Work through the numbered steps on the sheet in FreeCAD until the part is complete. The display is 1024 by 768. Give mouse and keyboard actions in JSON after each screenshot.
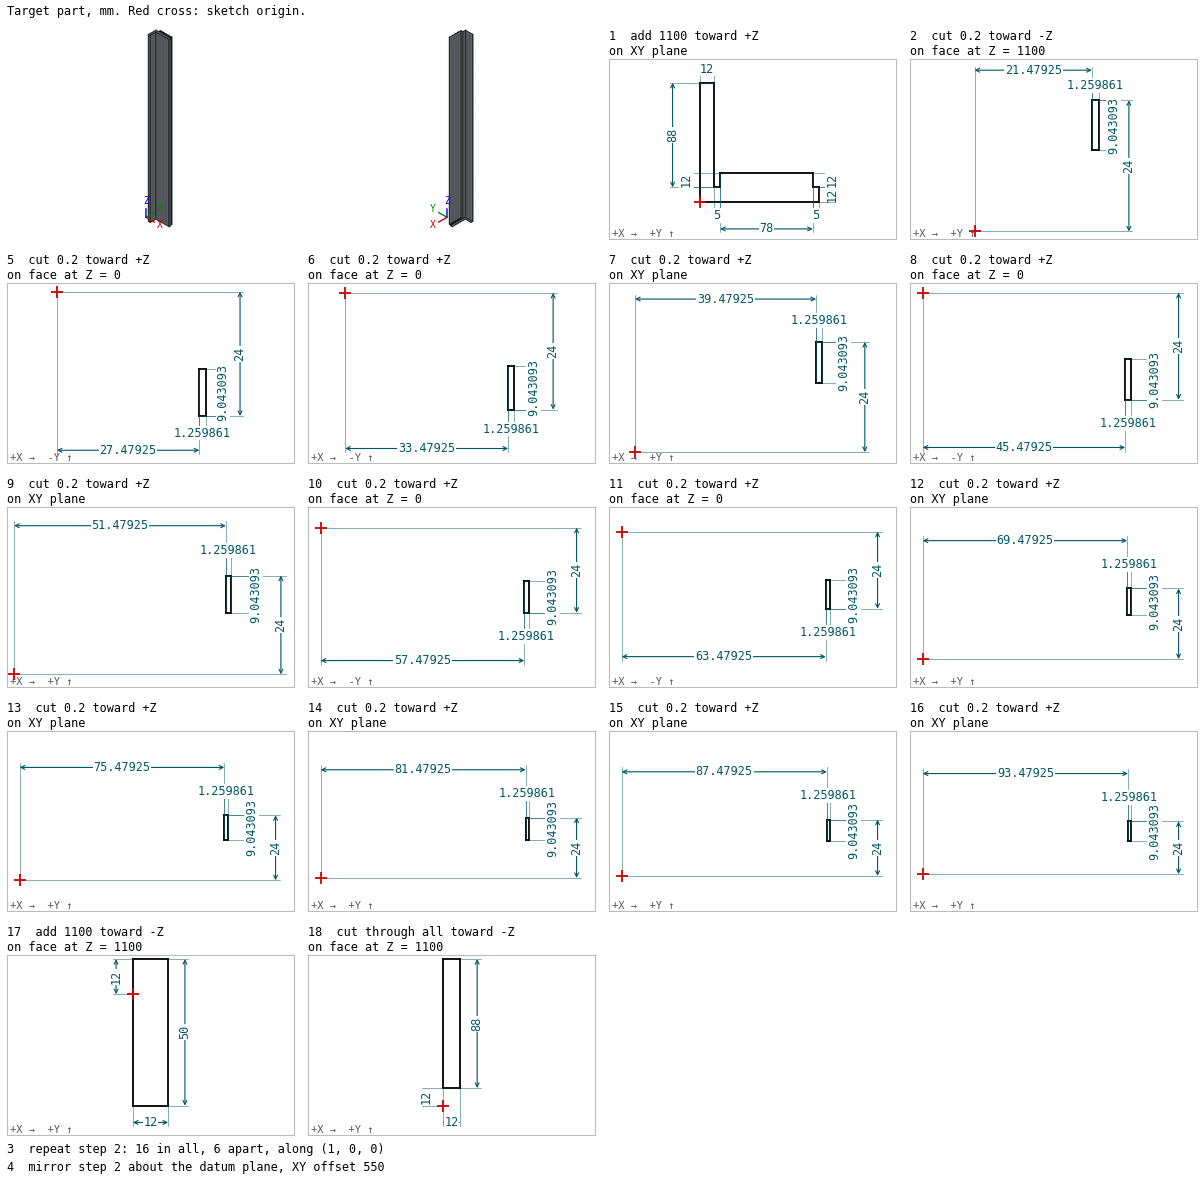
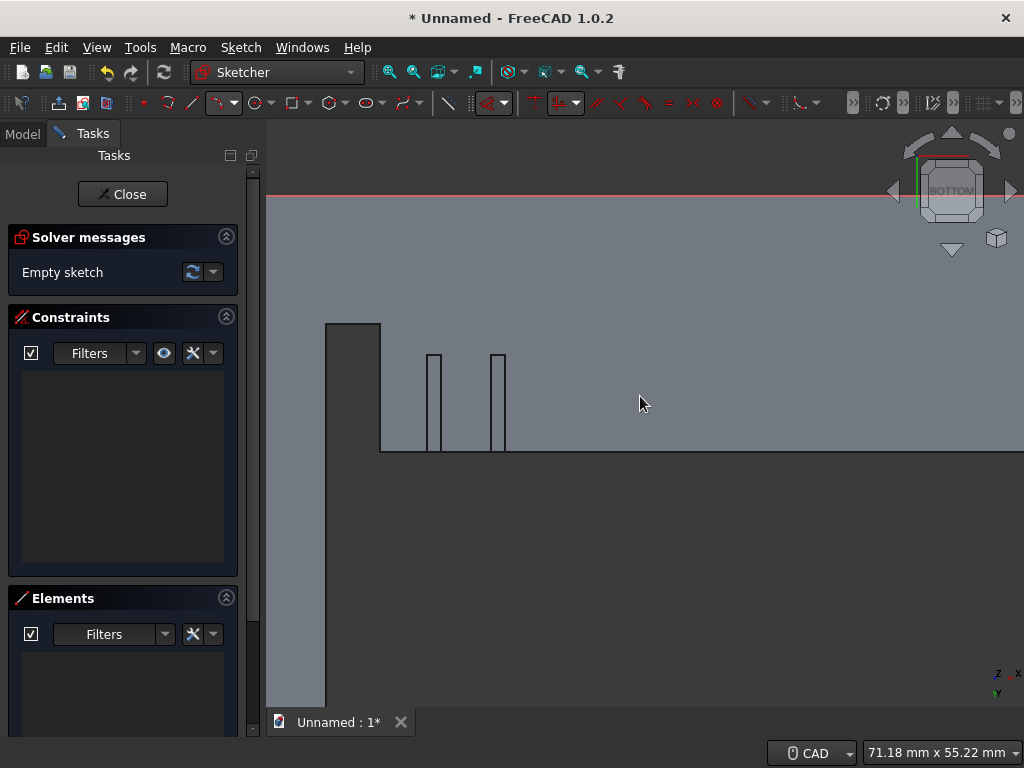
{"action": "scroll", "coordinate": [557, 400], "scroll_direction": "up", "scroll_amount": 7}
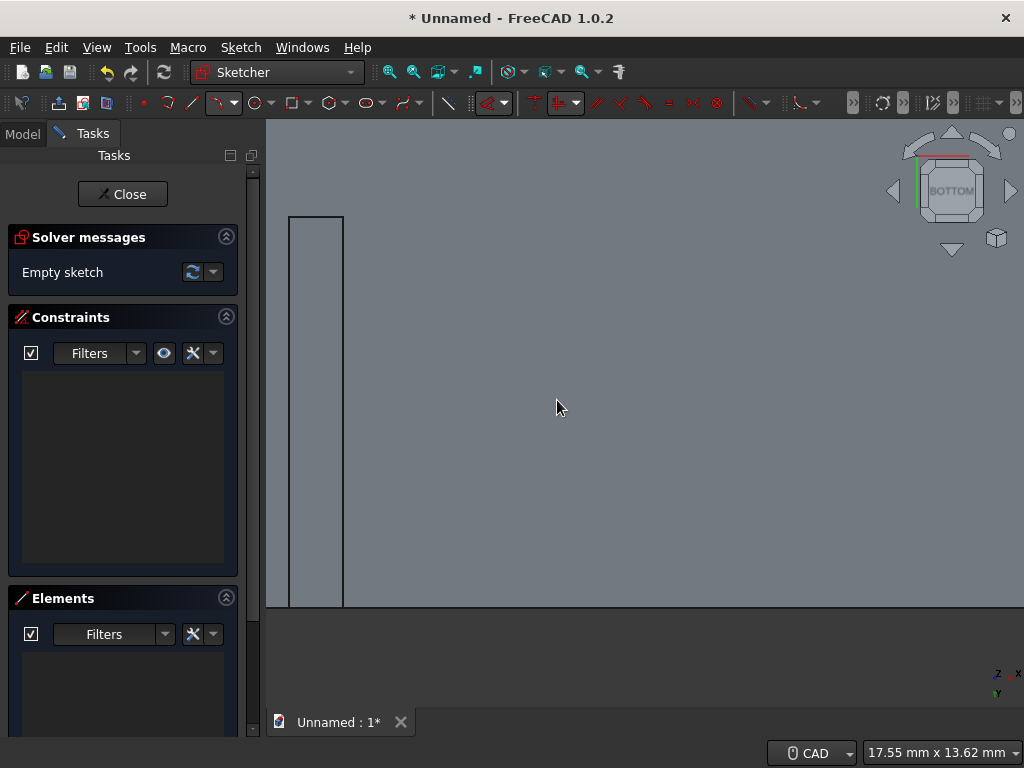
{"action": "key", "text": "g r"}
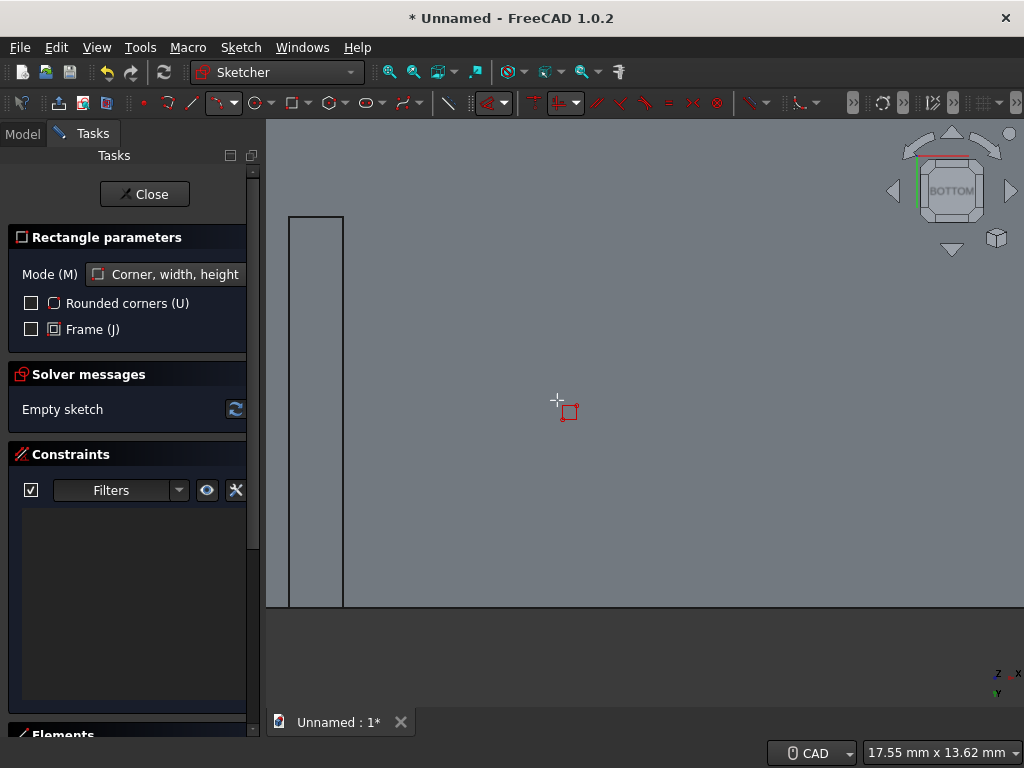
{"action": "left_click", "coordinate": [548, 217]}
{"action": "mouse_move", "coordinate": [602, 608]}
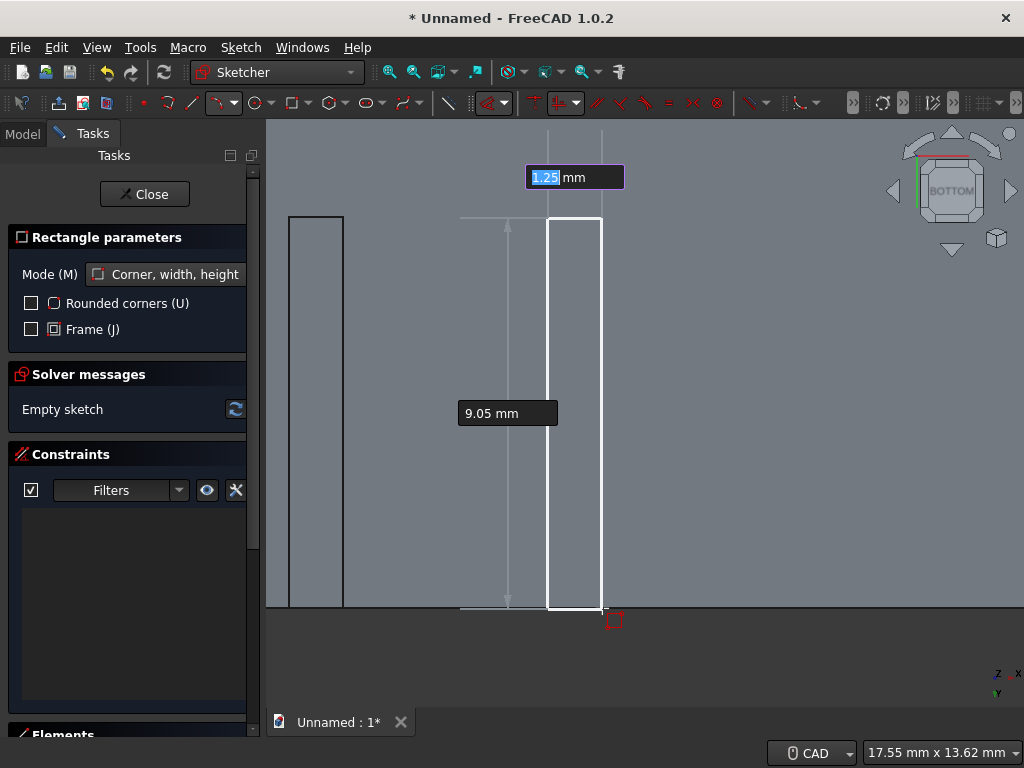
{"action": "type", "text": "1.259861"}
{"action": "key", "text": "Tab"}
{"action": "type", "text": "9.043093"}
{"action": "key", "text": "Return"}
{"action": "key", "text": "Escape"}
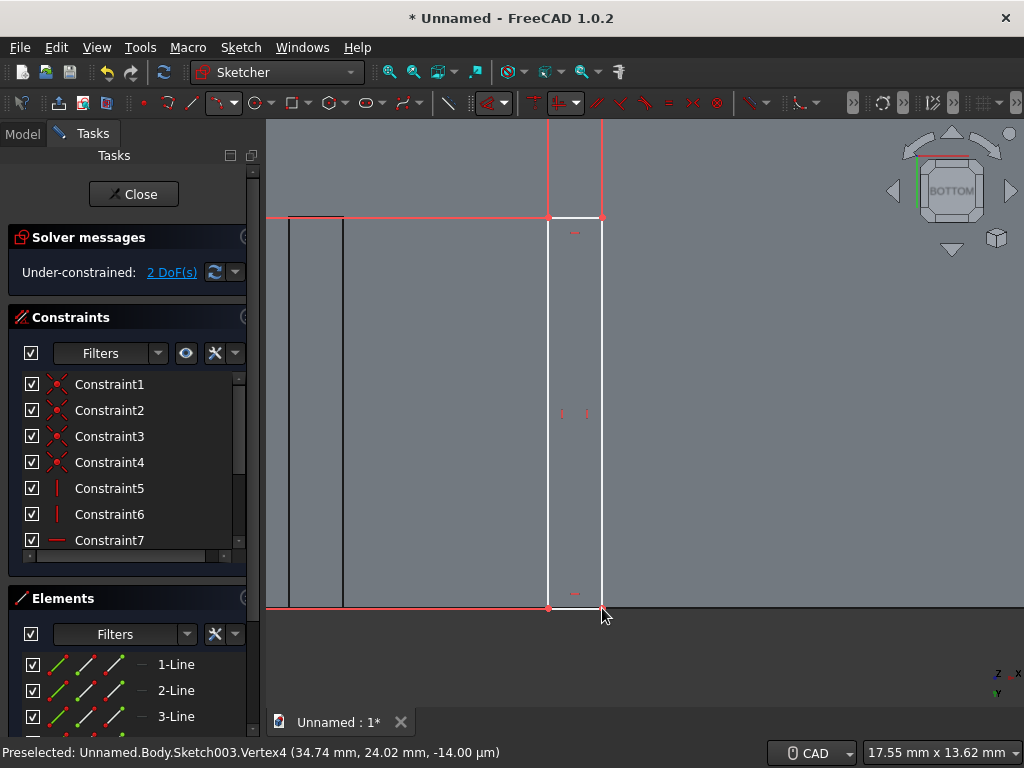
{"action": "left_click", "coordinate": [548, 609]}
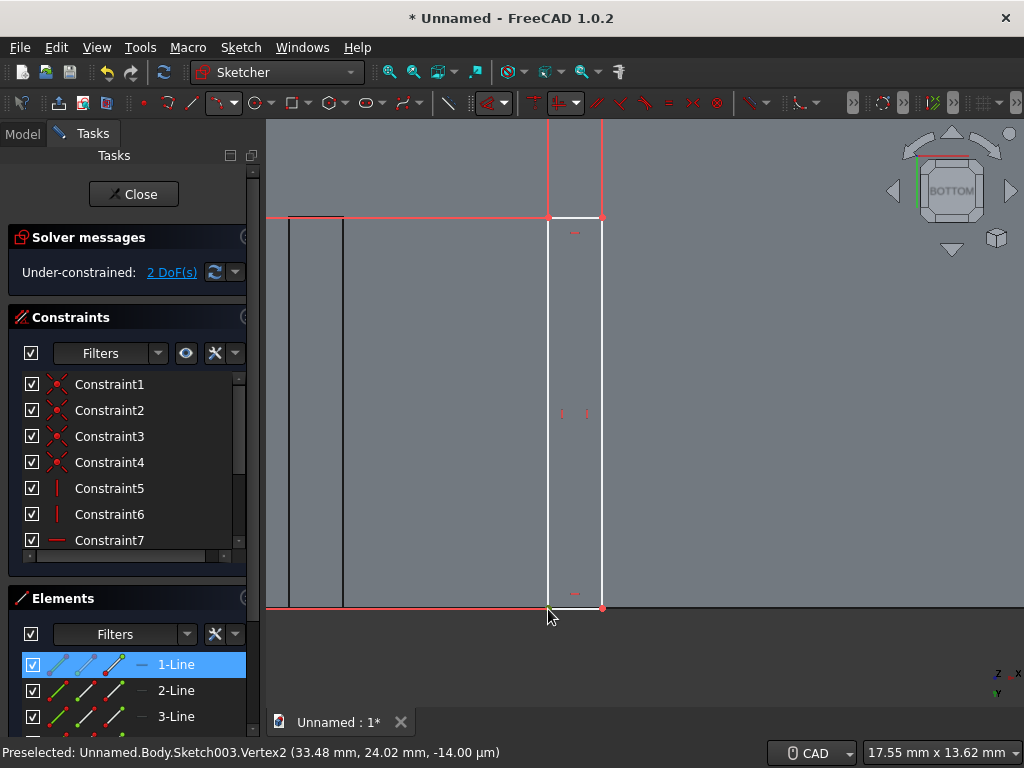
{"action": "left_click", "coordinate": [506, 104]}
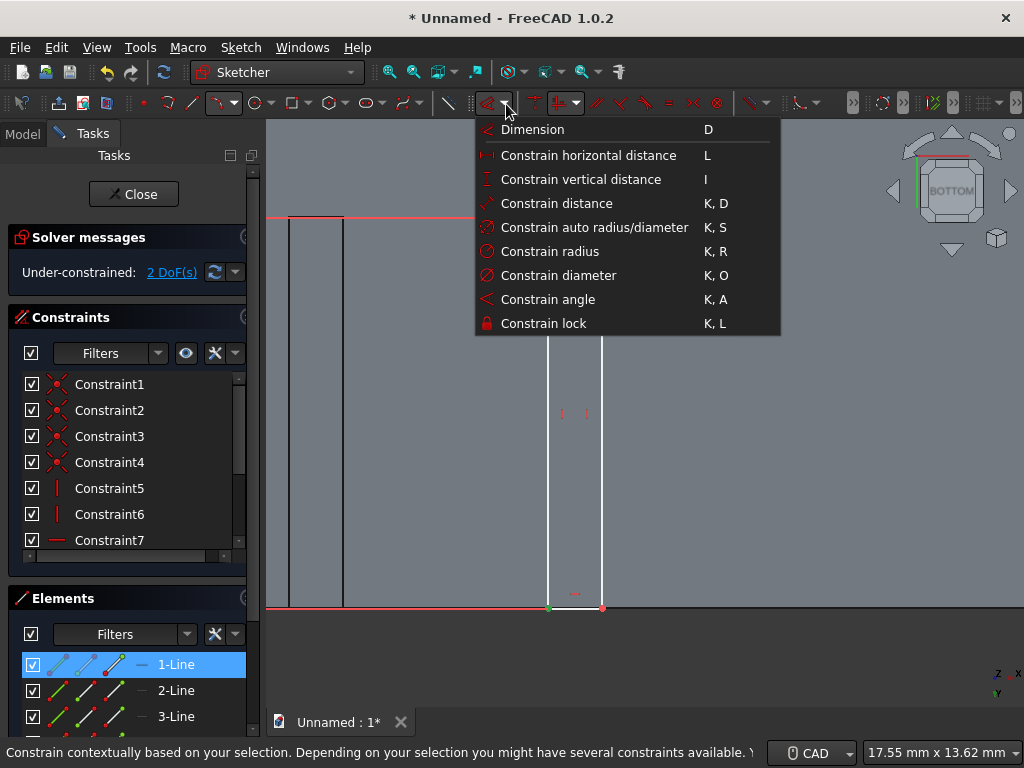
{"action": "left_click", "coordinate": [628, 179]}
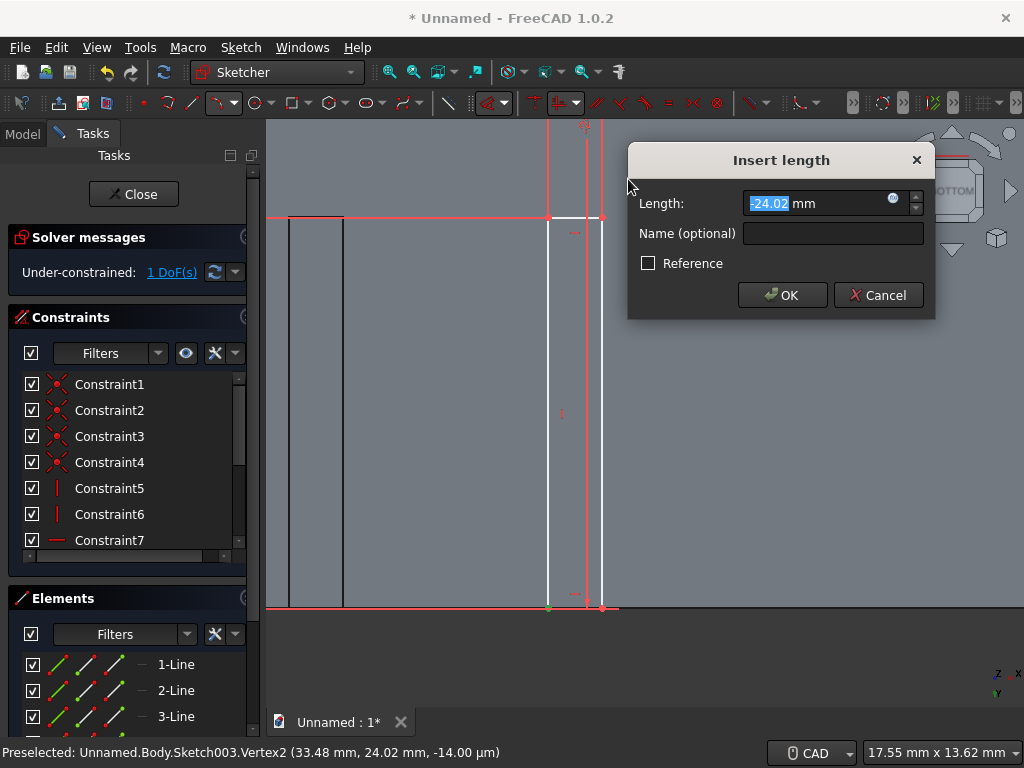
{"action": "type", "text": "-24"}
{"action": "key", "text": "Return"}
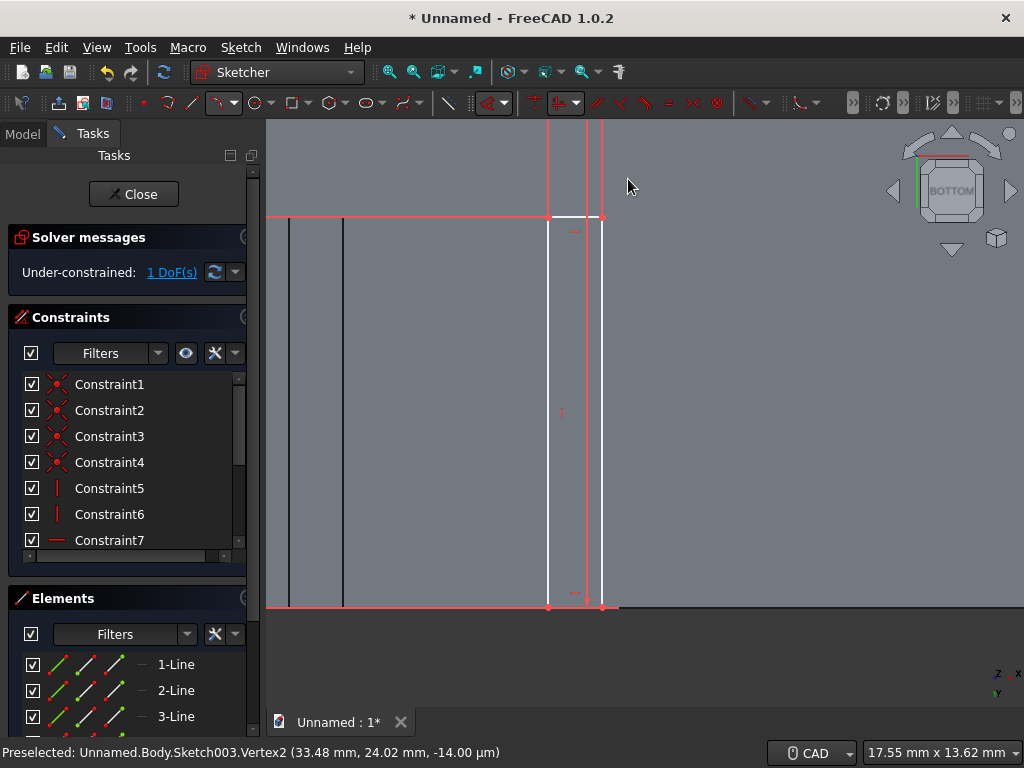
{"action": "left_click", "coordinate": [548, 217]}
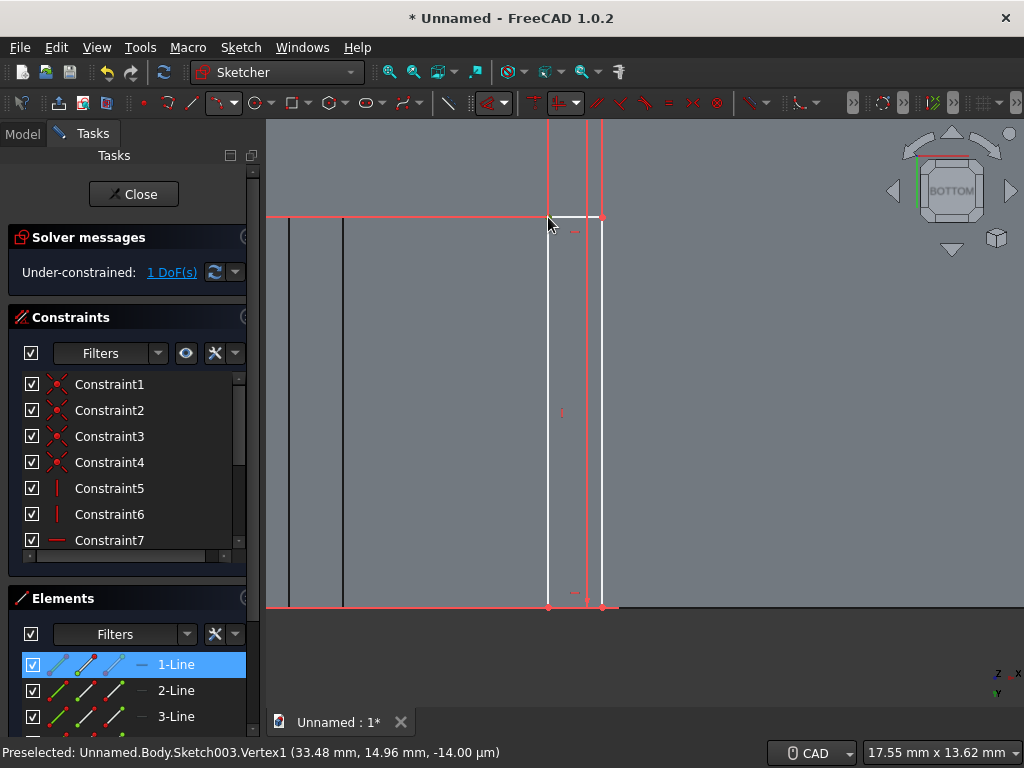
{"action": "key", "text": "l"}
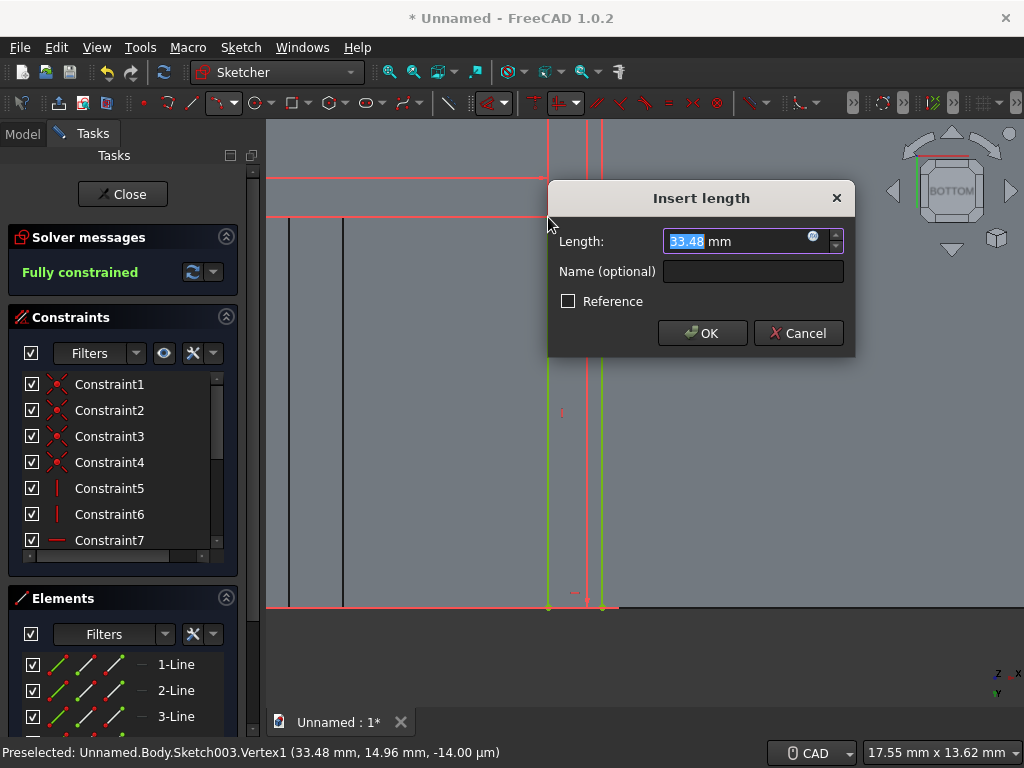
{"action": "type", "text": "33.47925"}
{"action": "key", "text": "Return"}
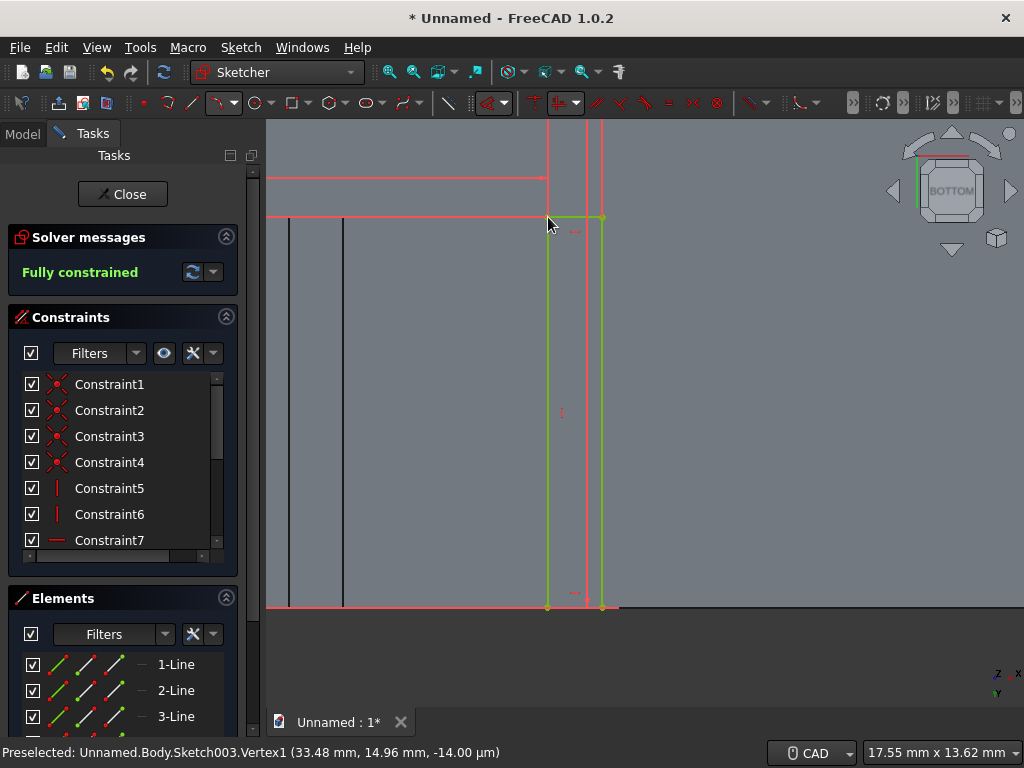
{"action": "left_click", "coordinate": [123, 194]}